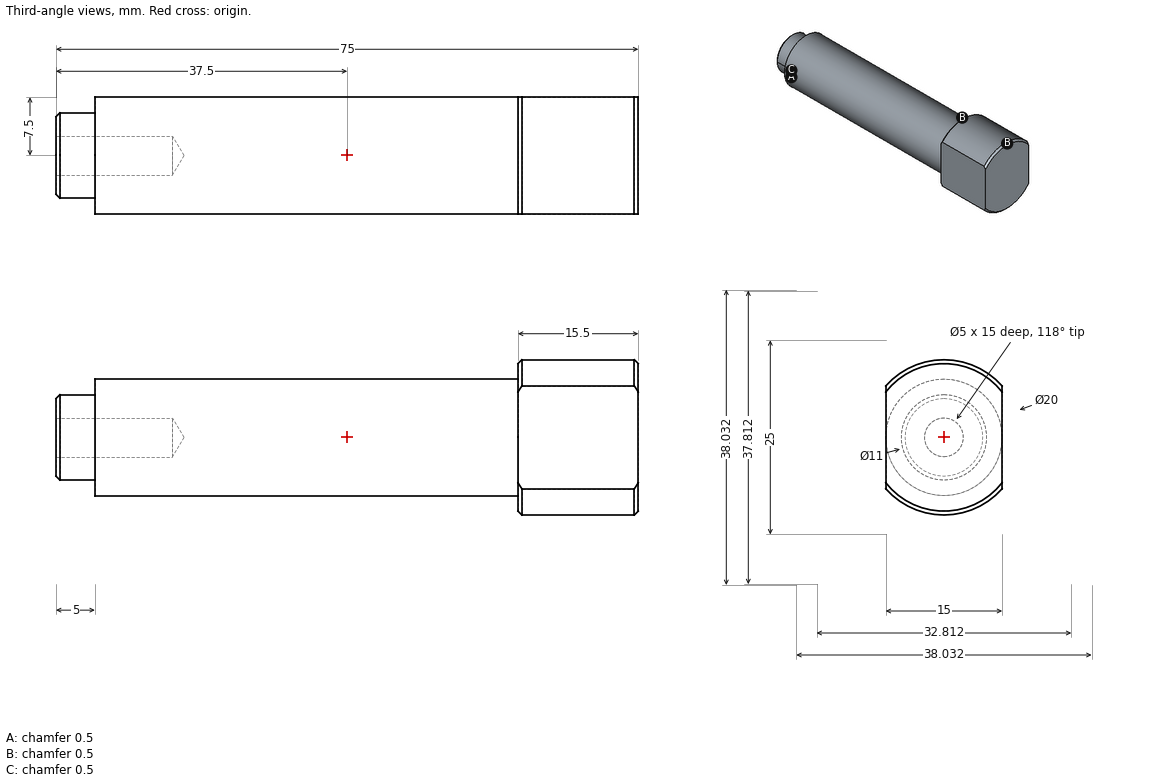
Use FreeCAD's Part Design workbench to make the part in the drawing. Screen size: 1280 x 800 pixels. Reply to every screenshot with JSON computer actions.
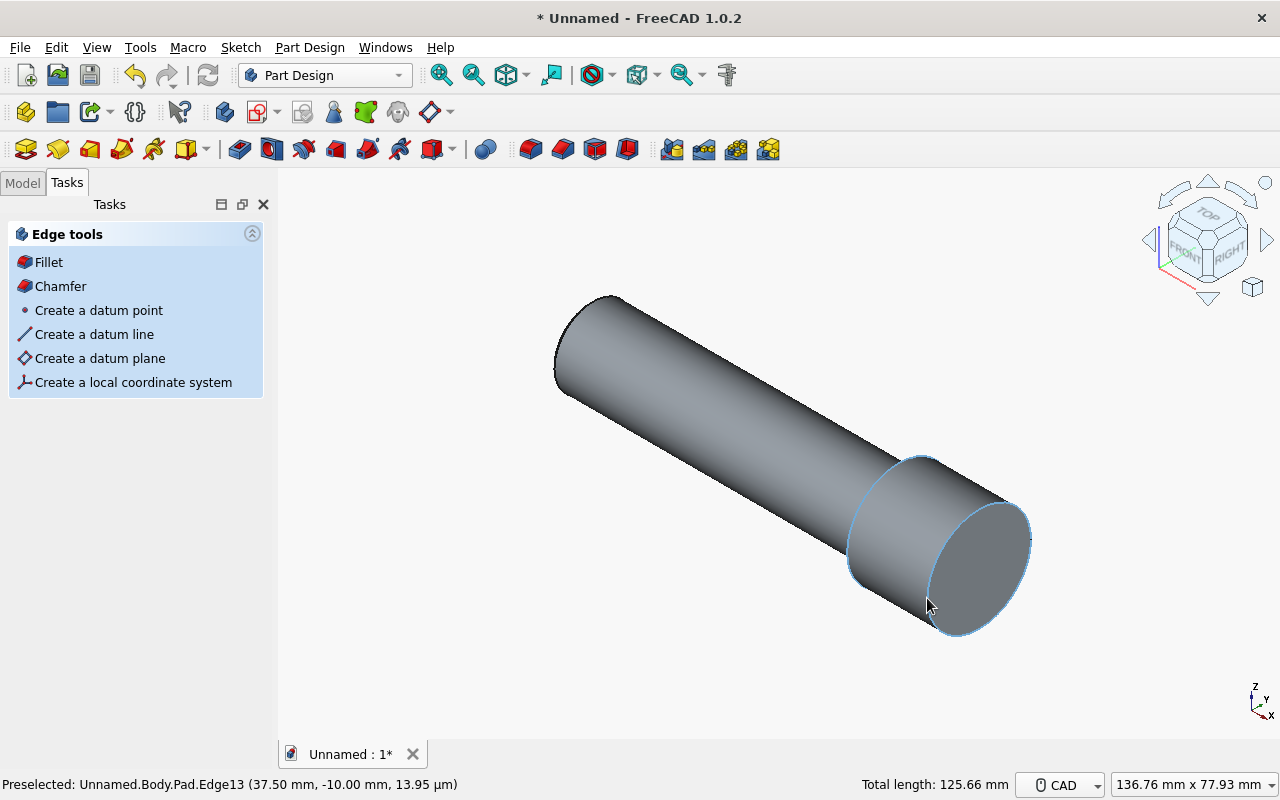
{"action": "left_click", "coordinate": [564, 150]}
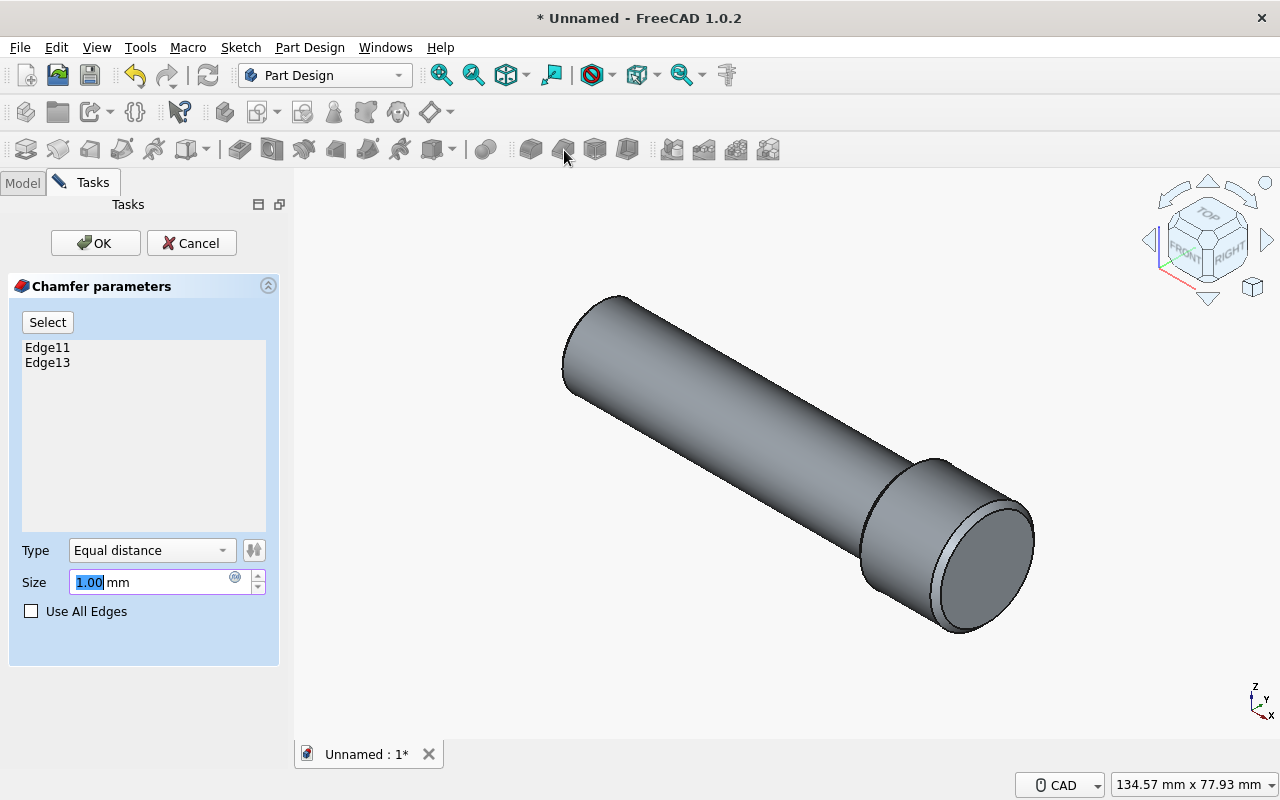
{"action": "type", "text": "0.5"}
{"action": "key", "text": "Tab"}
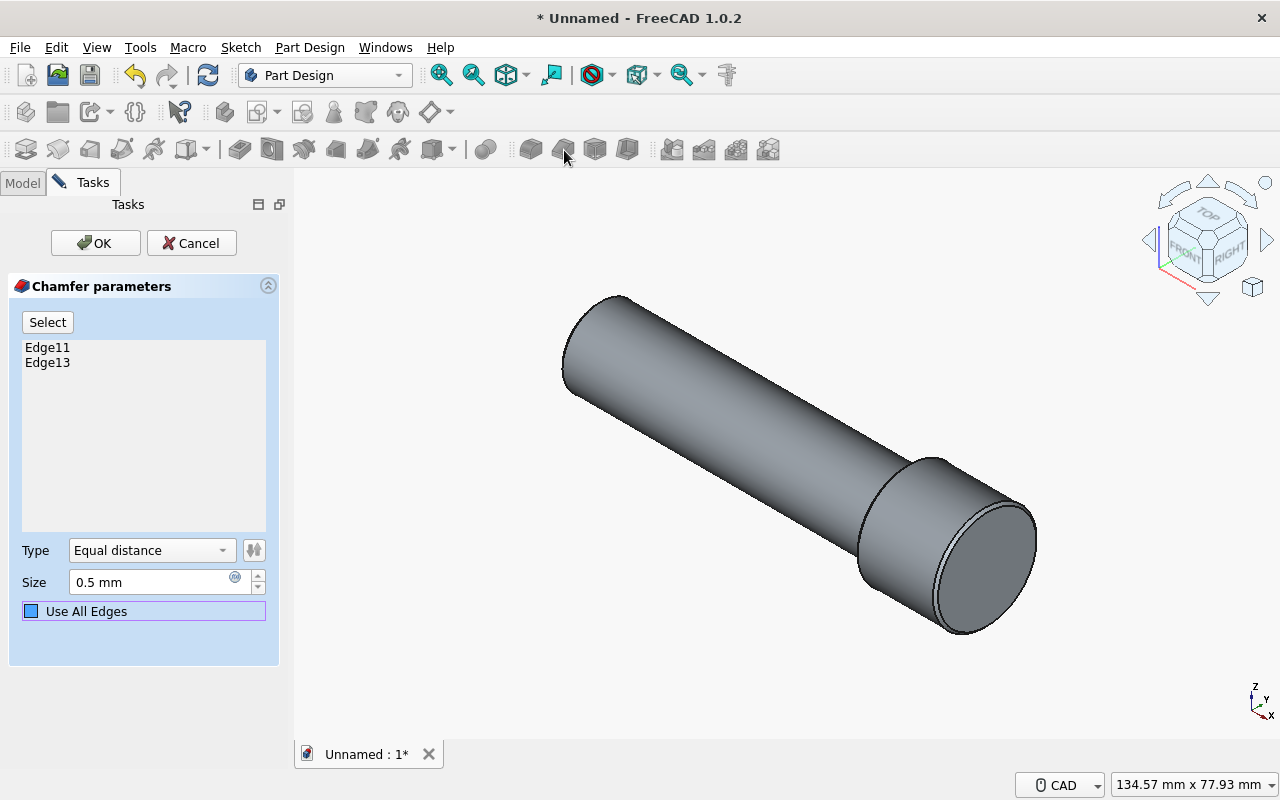
{"action": "left_click", "coordinate": [96, 243]}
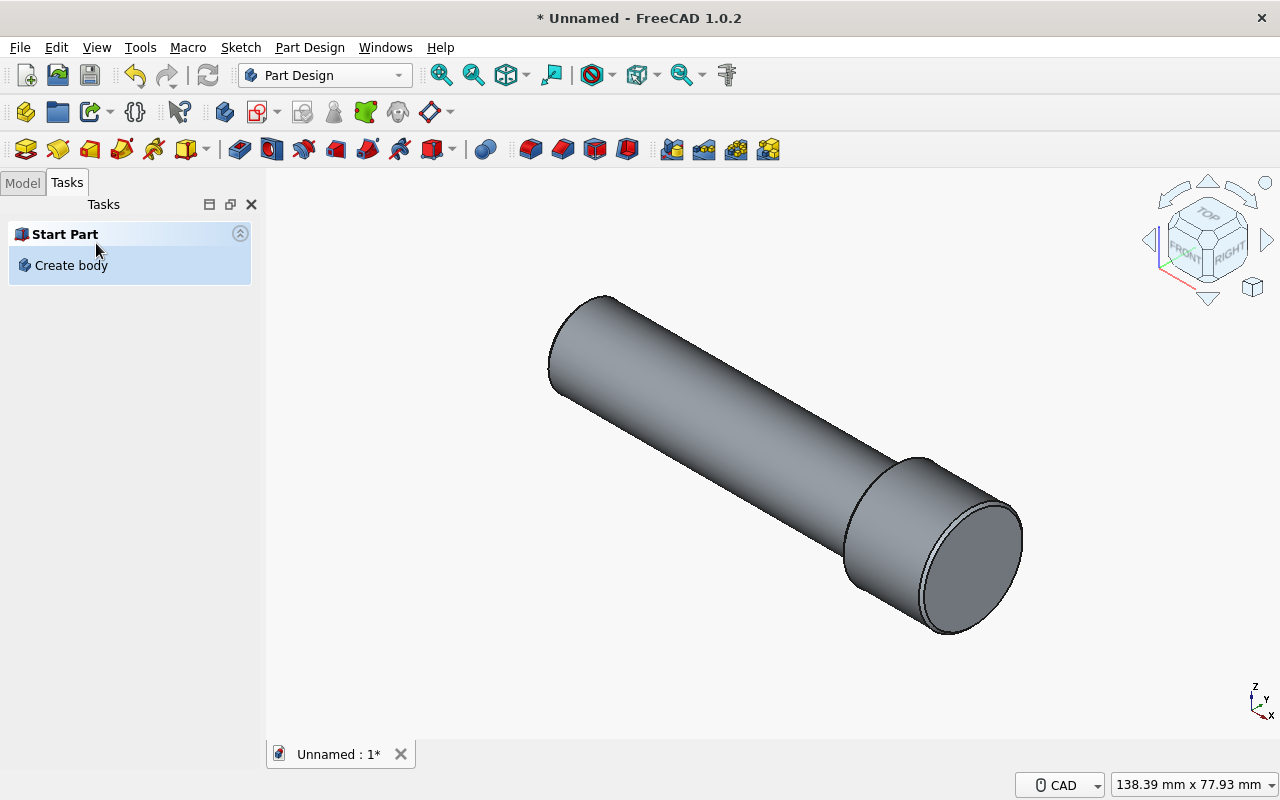
{"action": "key", "text": "6"}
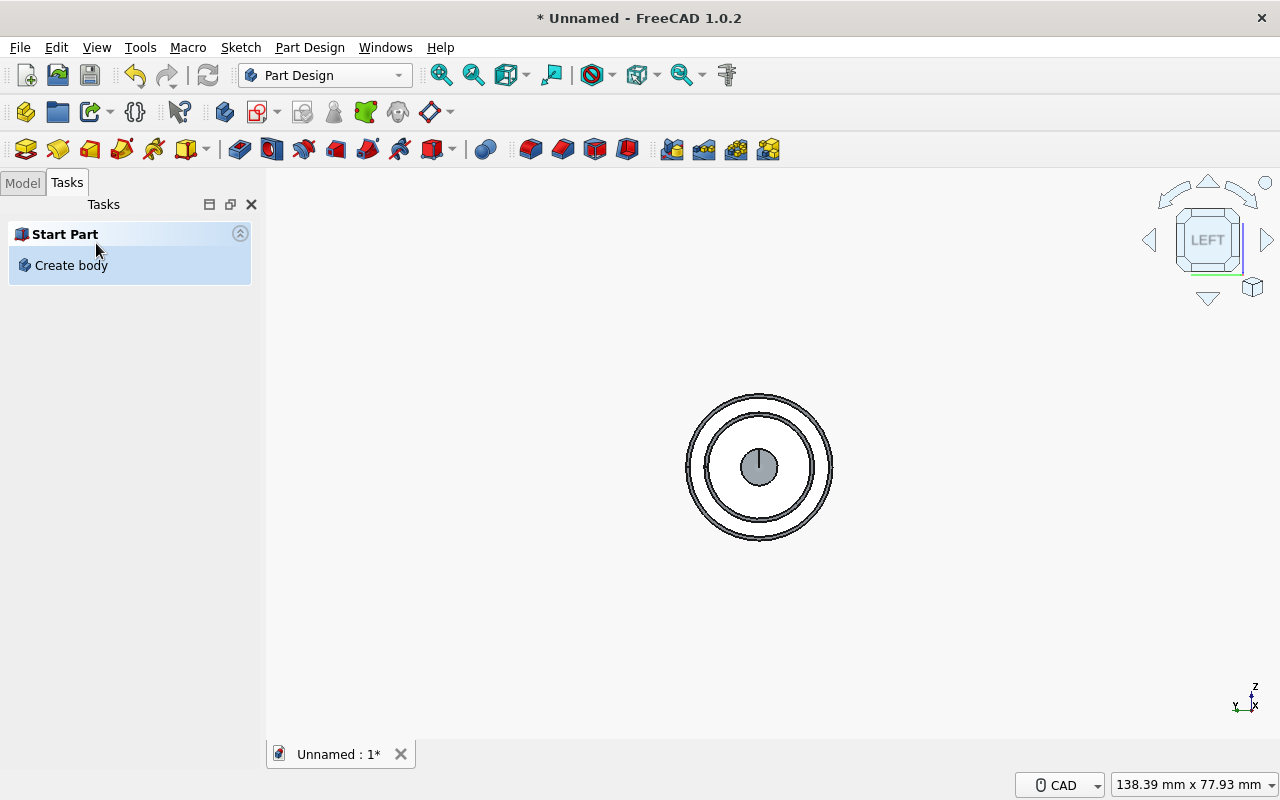
{"action": "key", "text": "v f"}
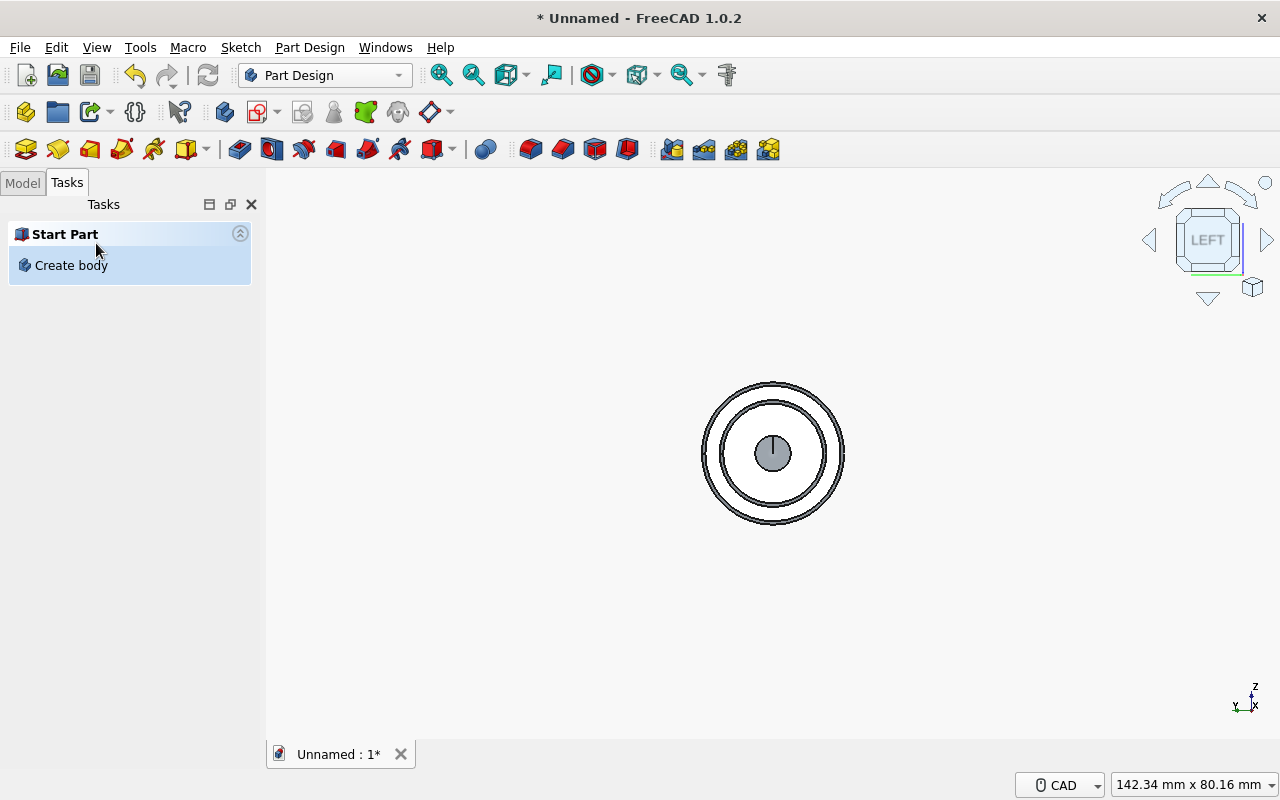
{"action": "scroll", "coordinate": [831, 472], "scroll_direction": "up", "scroll_amount": 4}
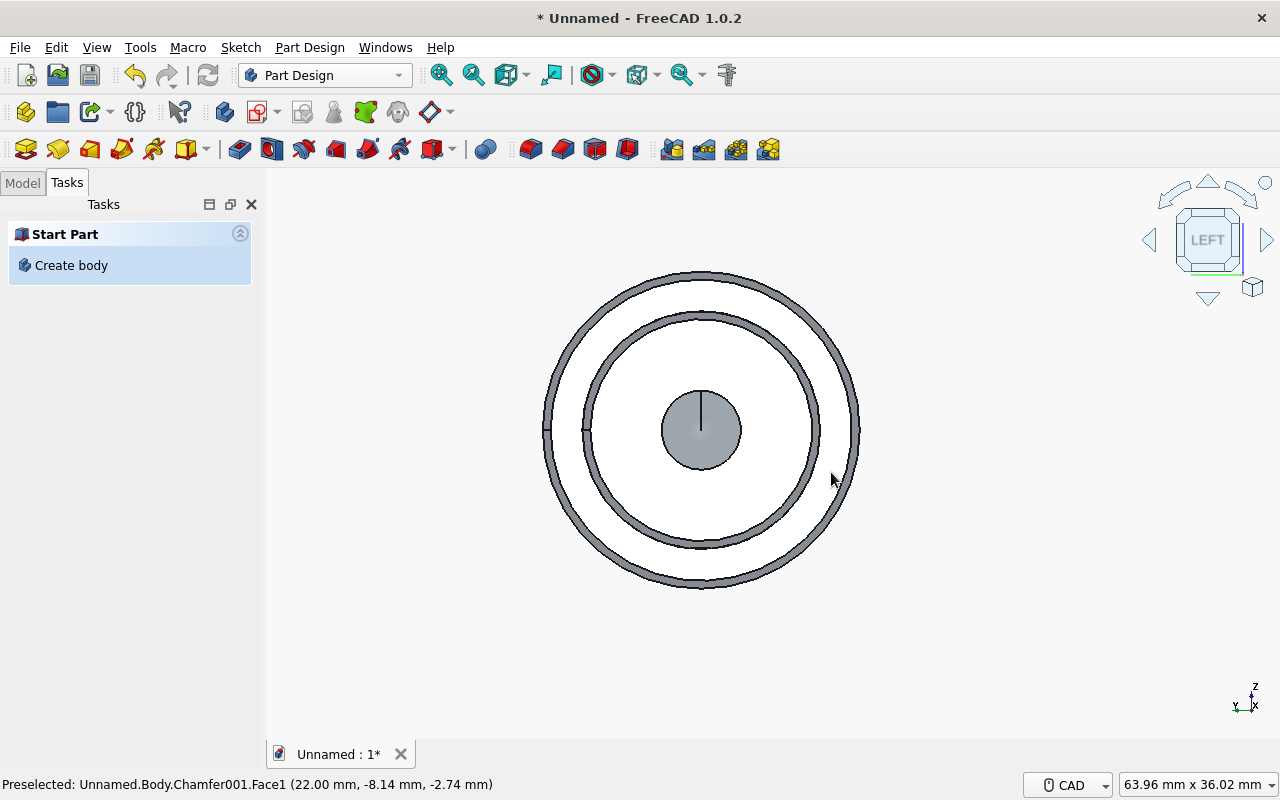
{"action": "left_click", "coordinate": [830, 472]}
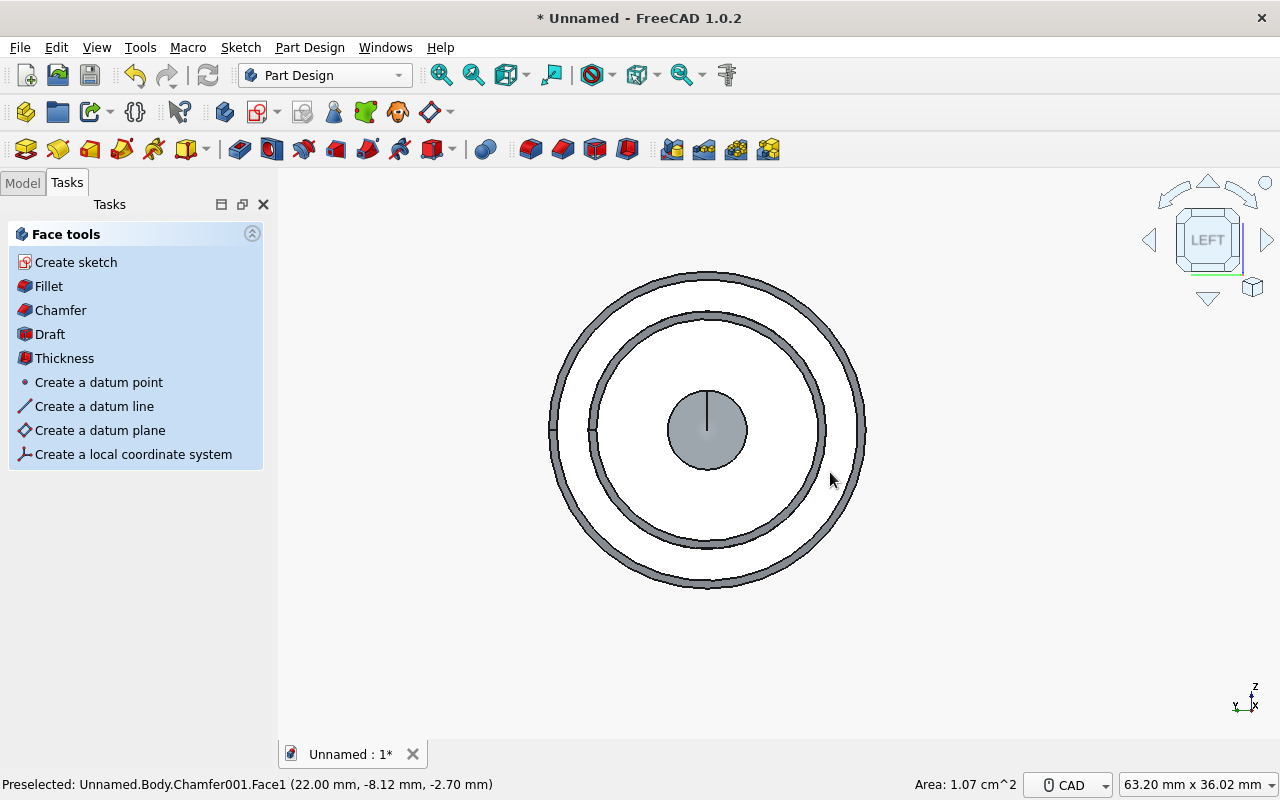
{"action": "left_click", "coordinate": [258, 112]}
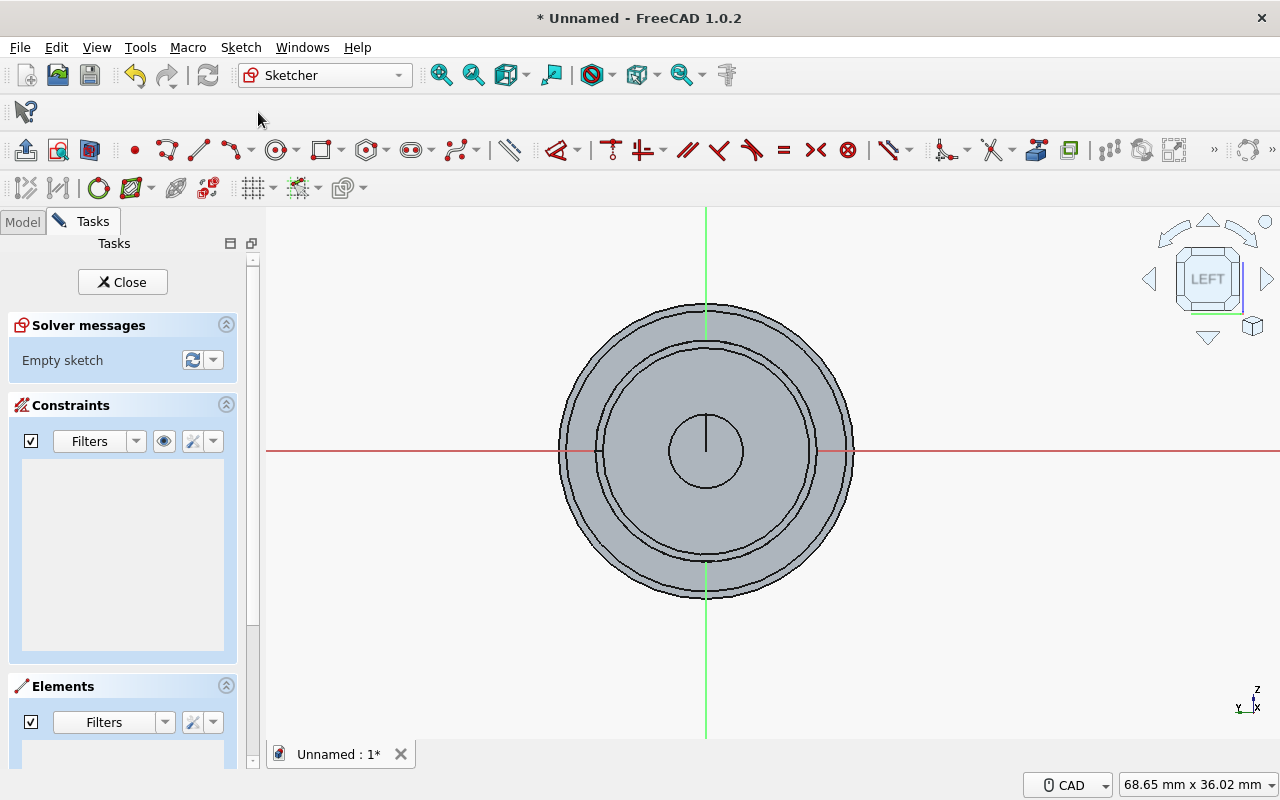
{"action": "left_click", "coordinate": [90, 150]}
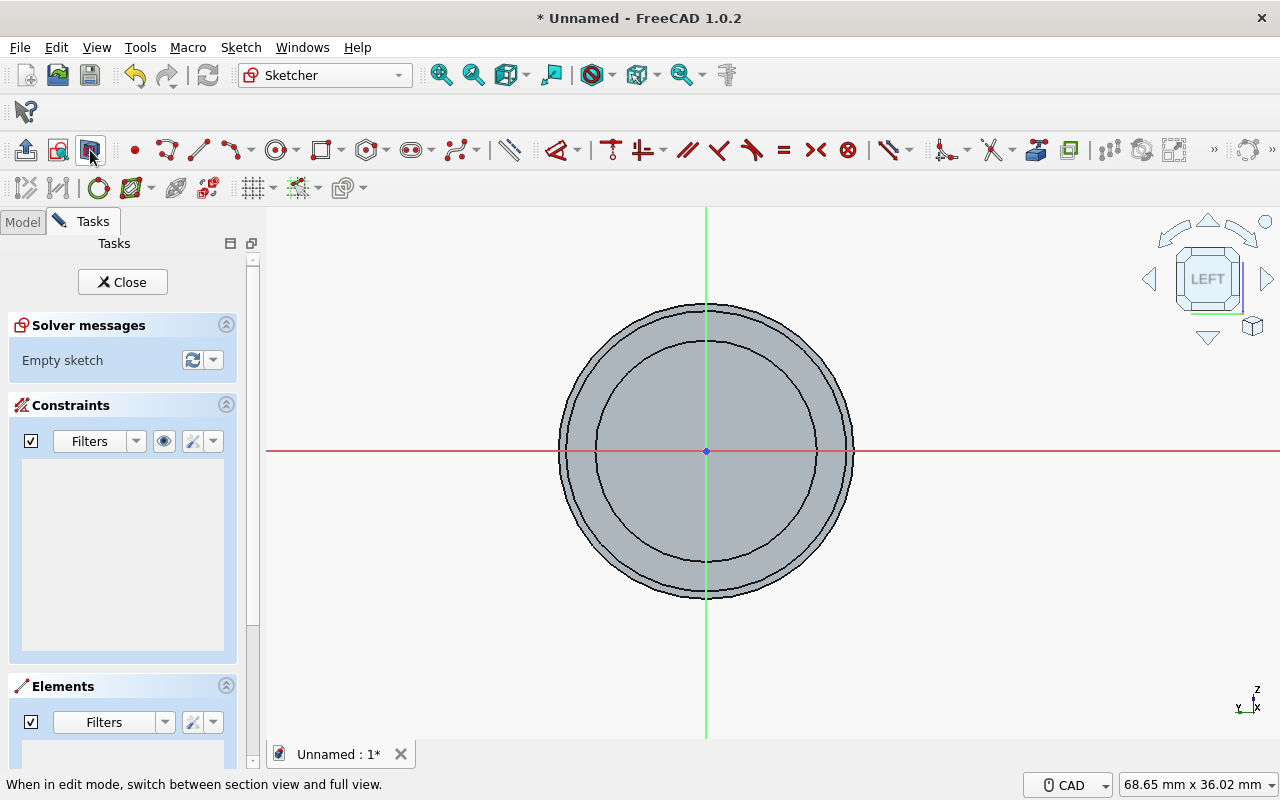
{"action": "scroll", "coordinate": [703, 499], "scroll_direction": "down", "scroll_amount": 3}